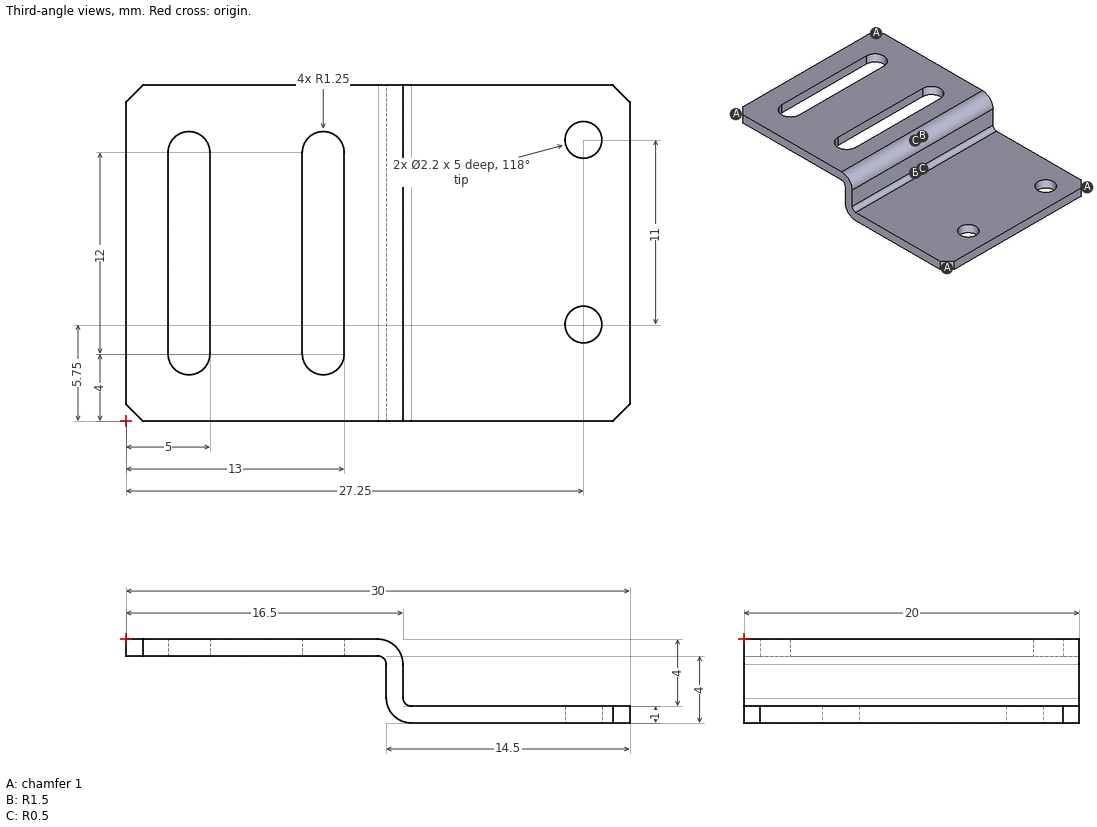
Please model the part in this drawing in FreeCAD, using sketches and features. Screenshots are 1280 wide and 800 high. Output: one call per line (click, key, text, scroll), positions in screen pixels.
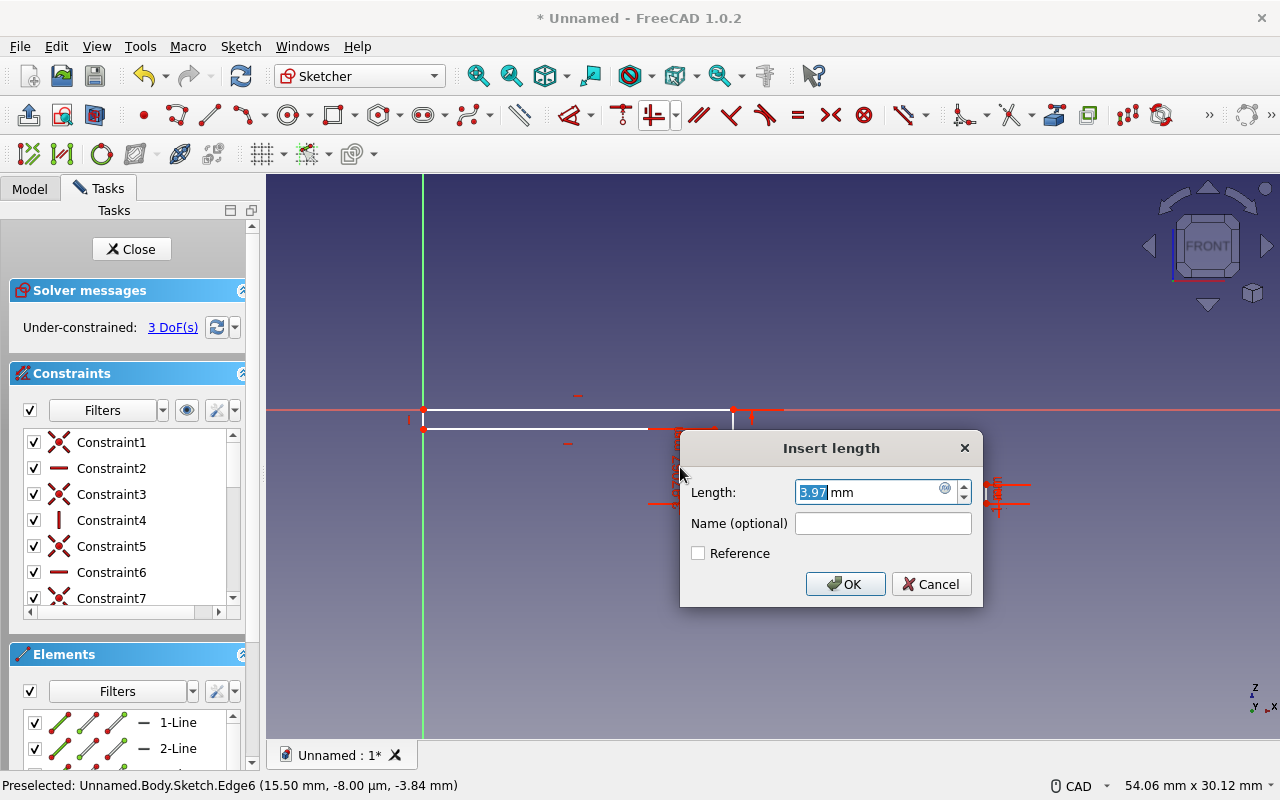
text(4)
key(Return)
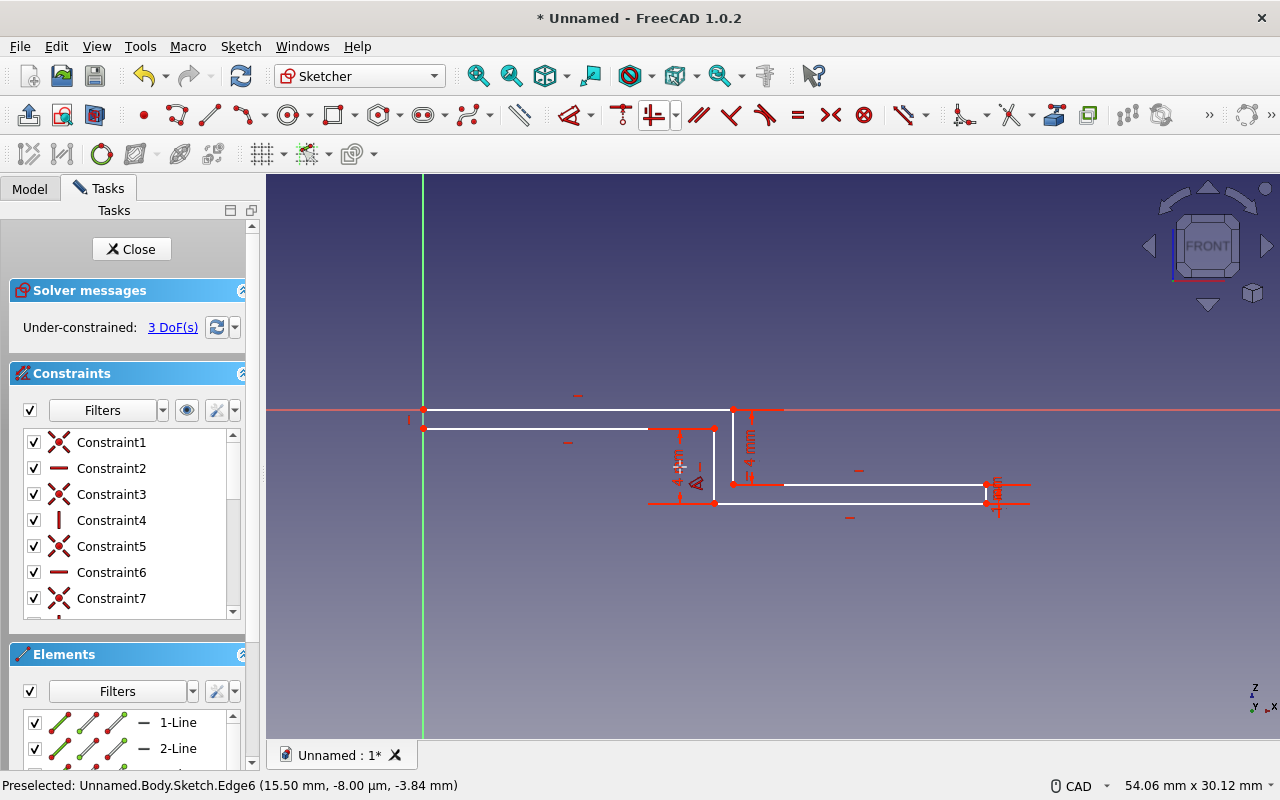
click(986, 485)
click(705, 376)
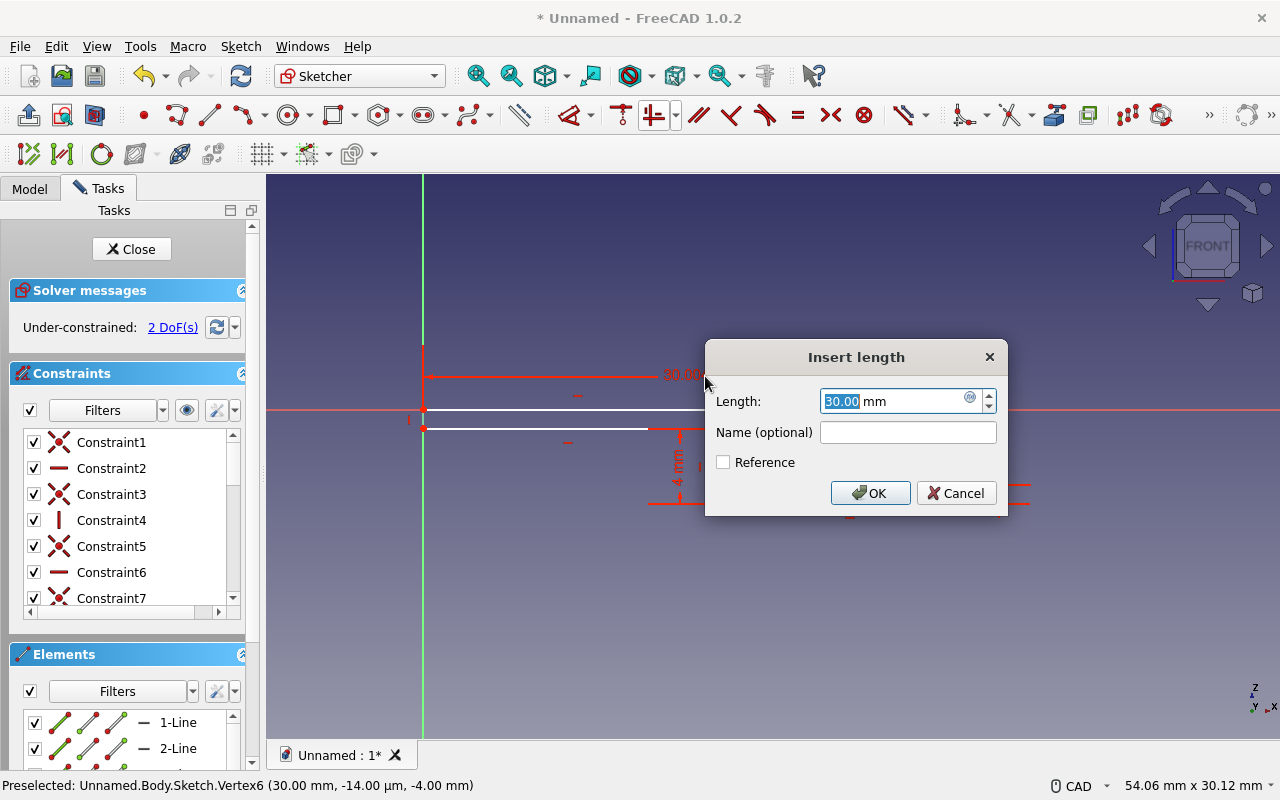
text(30)
key(Return)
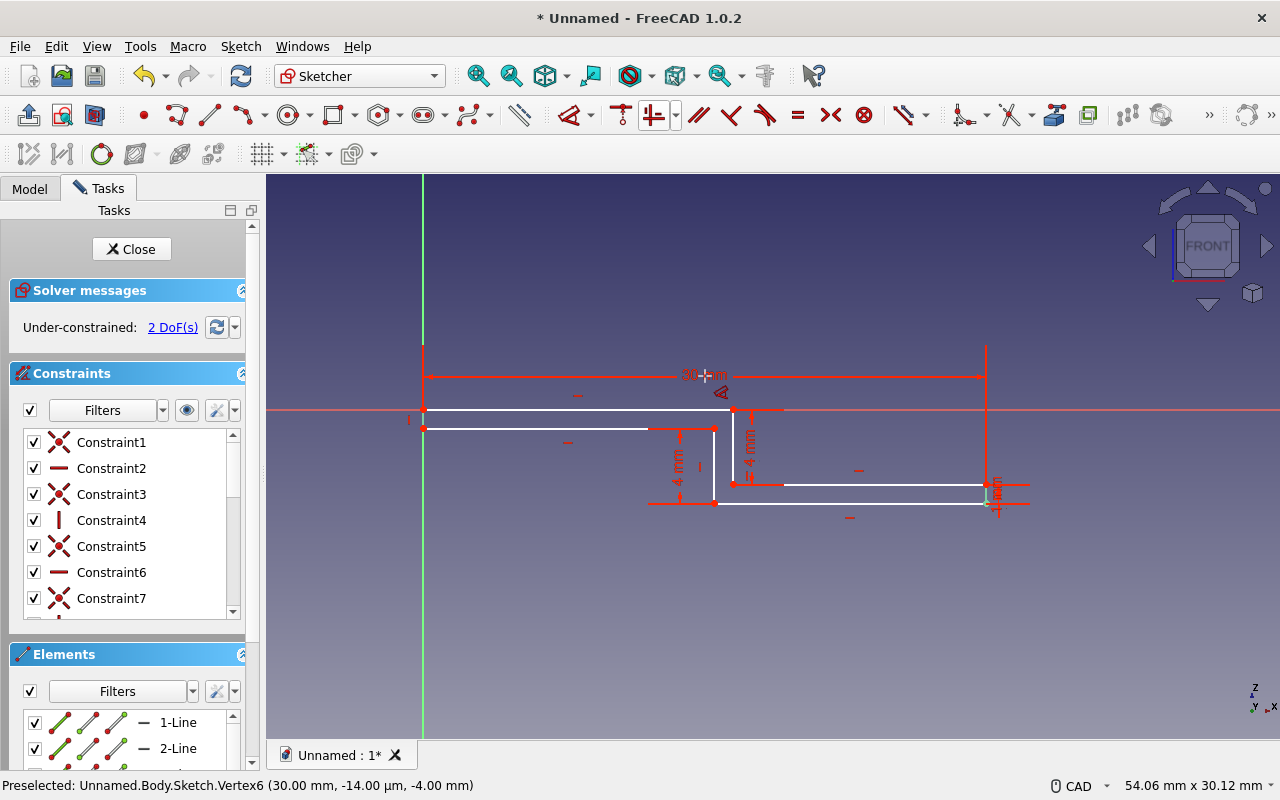
click(516, 410)
click(578, 376)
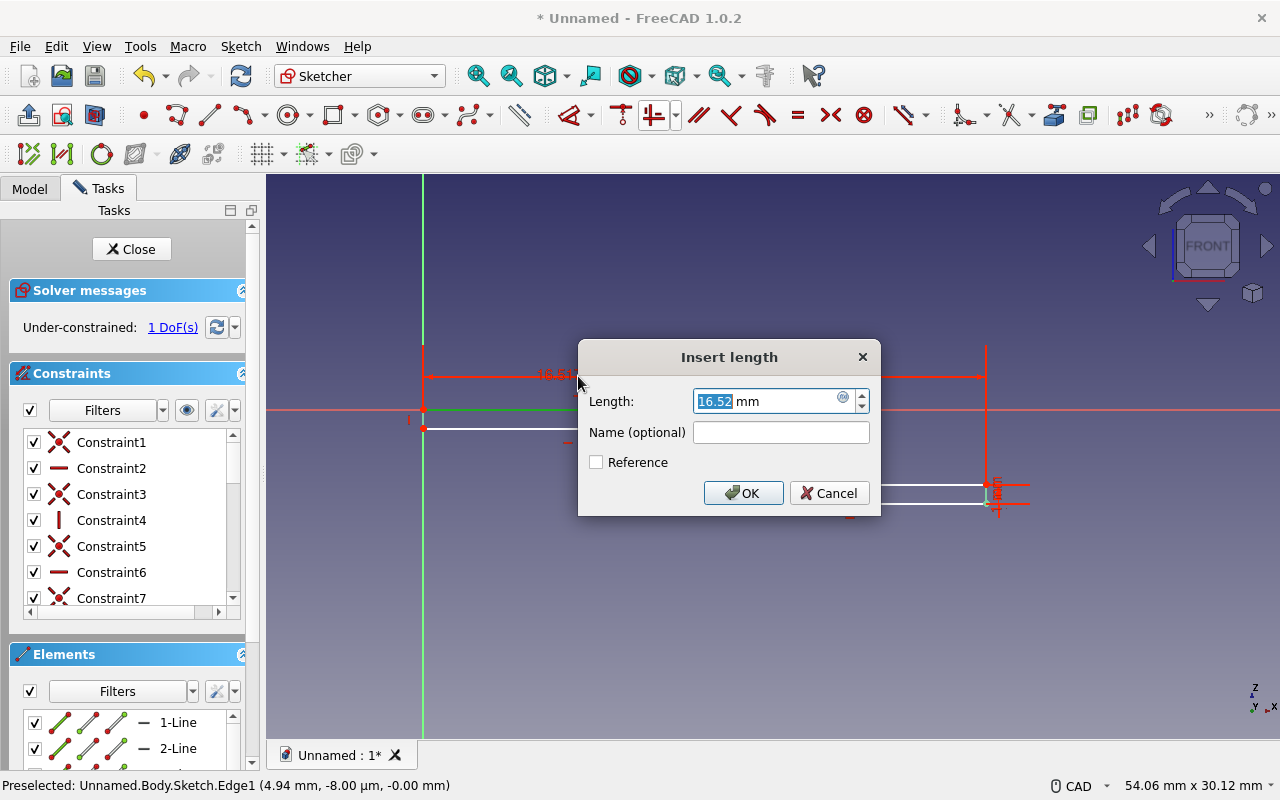
text(16.5)
key(Return)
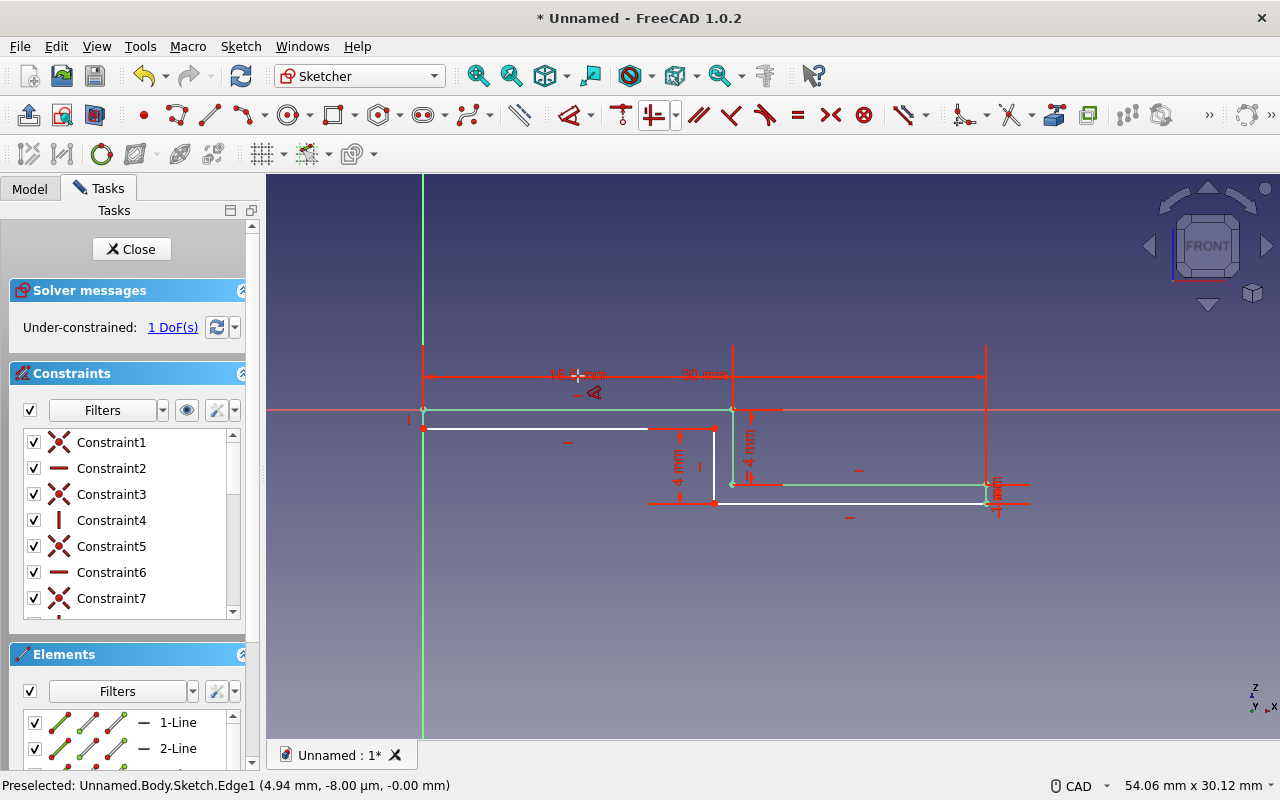
click(905, 504)
click(850, 538)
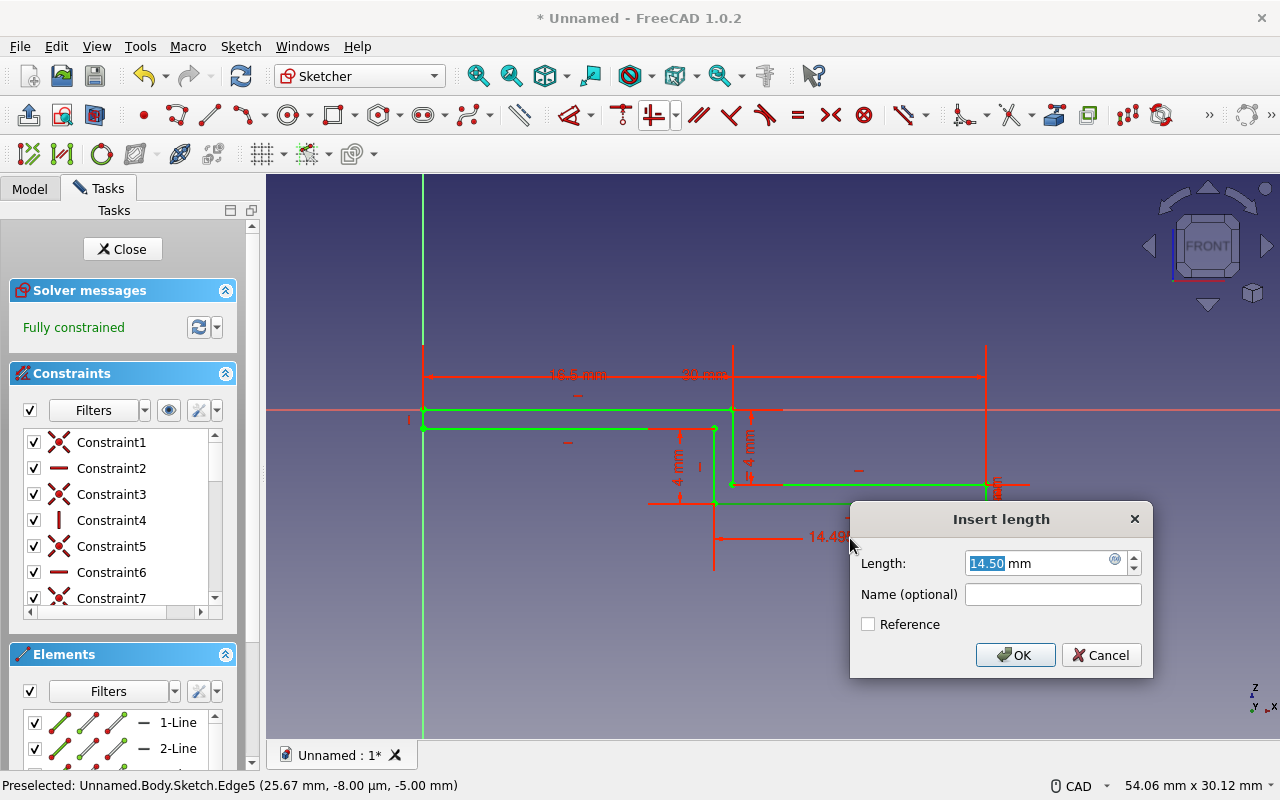
text(14.5)
key(Return)
key(Escape)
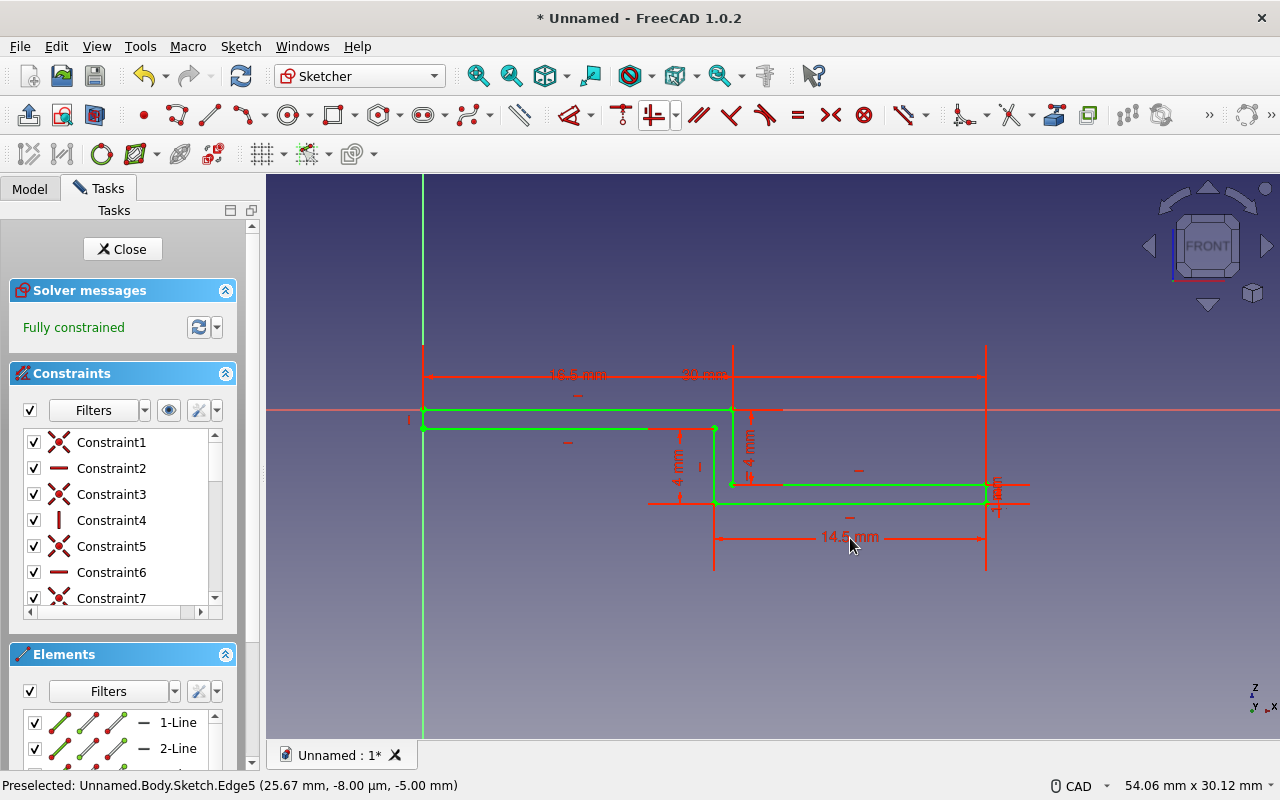
click(123, 249)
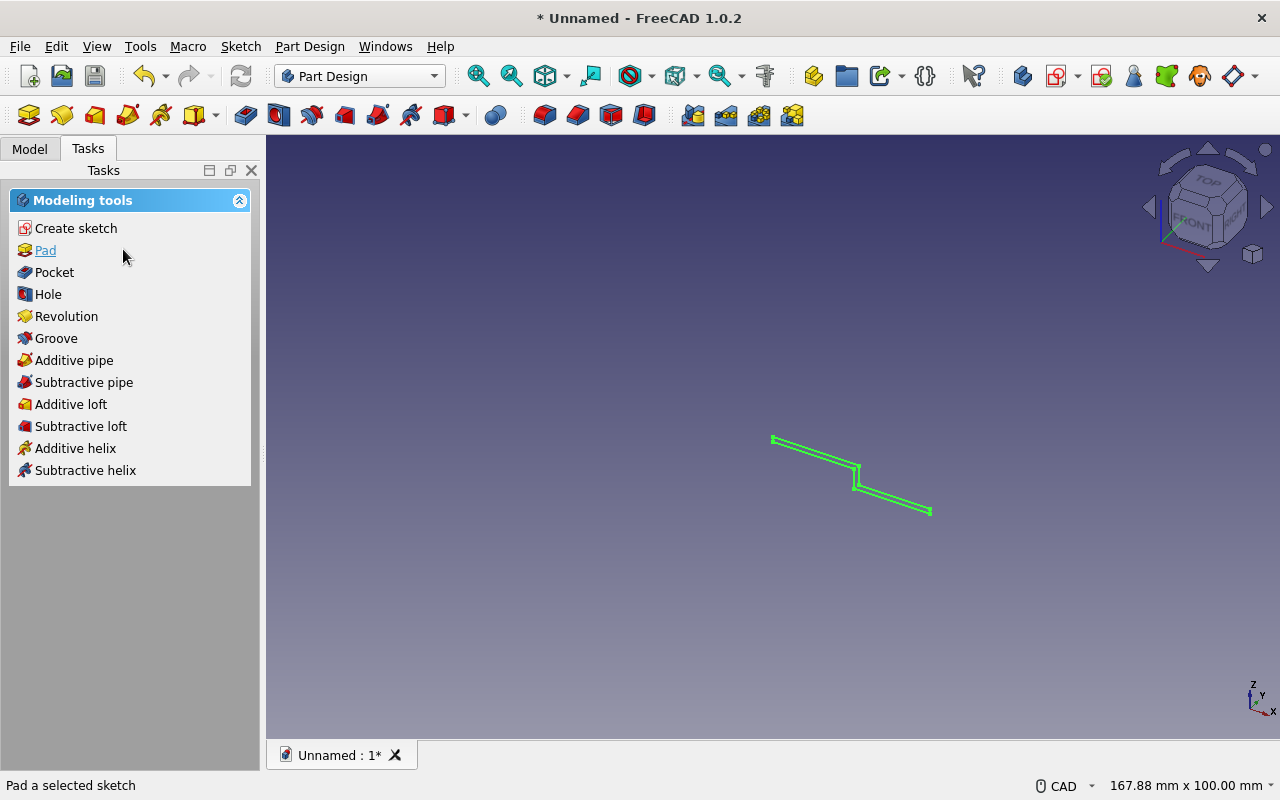
click(29, 116)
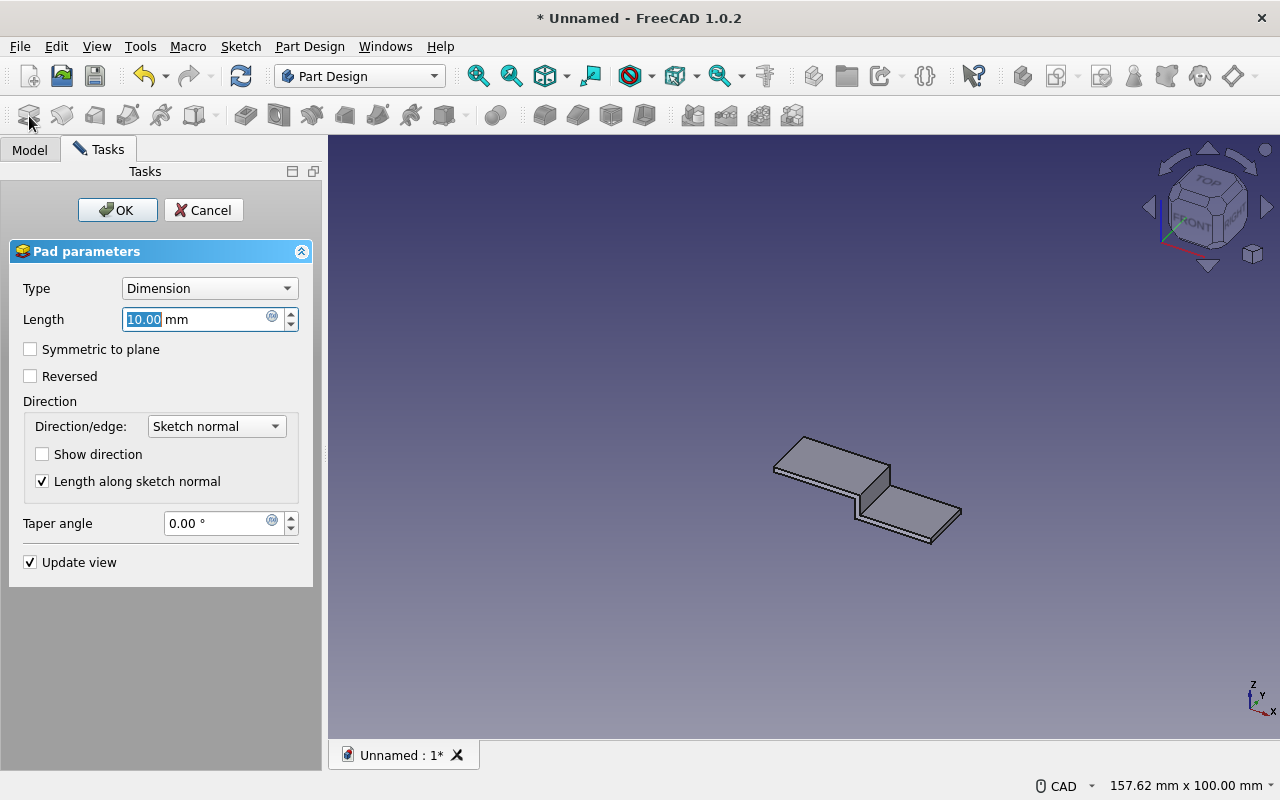
text(20)
key(Tab)